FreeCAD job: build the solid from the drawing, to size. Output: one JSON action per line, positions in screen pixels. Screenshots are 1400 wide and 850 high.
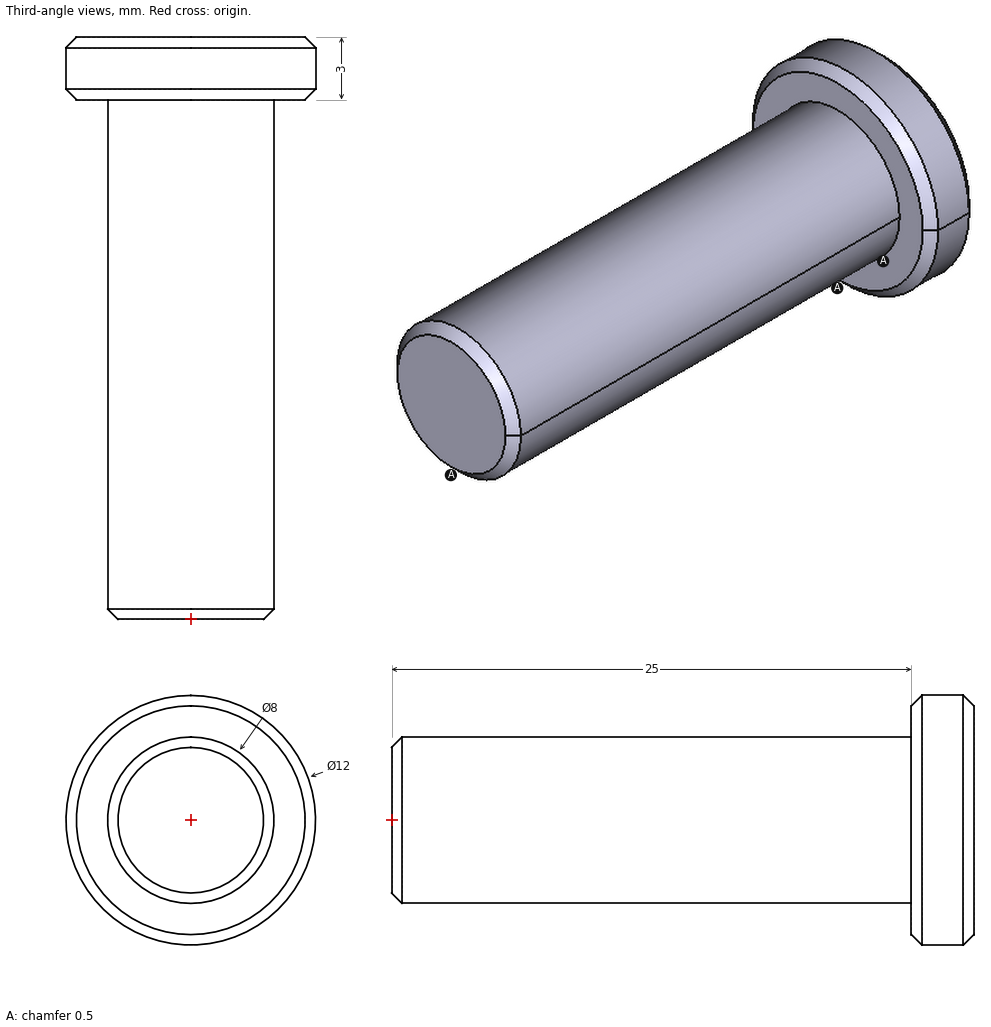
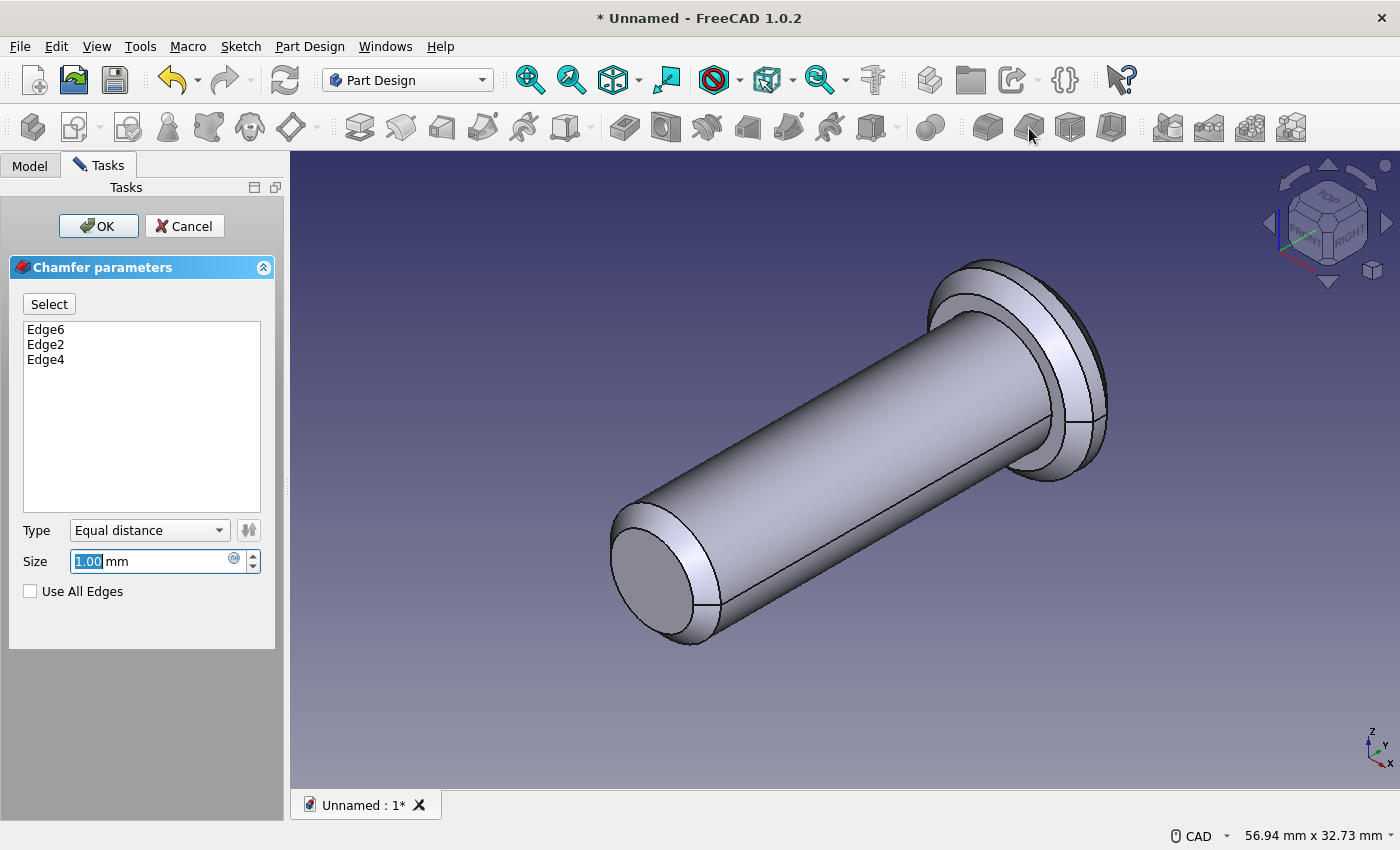
{"action": "type", "text": "0.5"}
{"action": "key", "text": "Tab"}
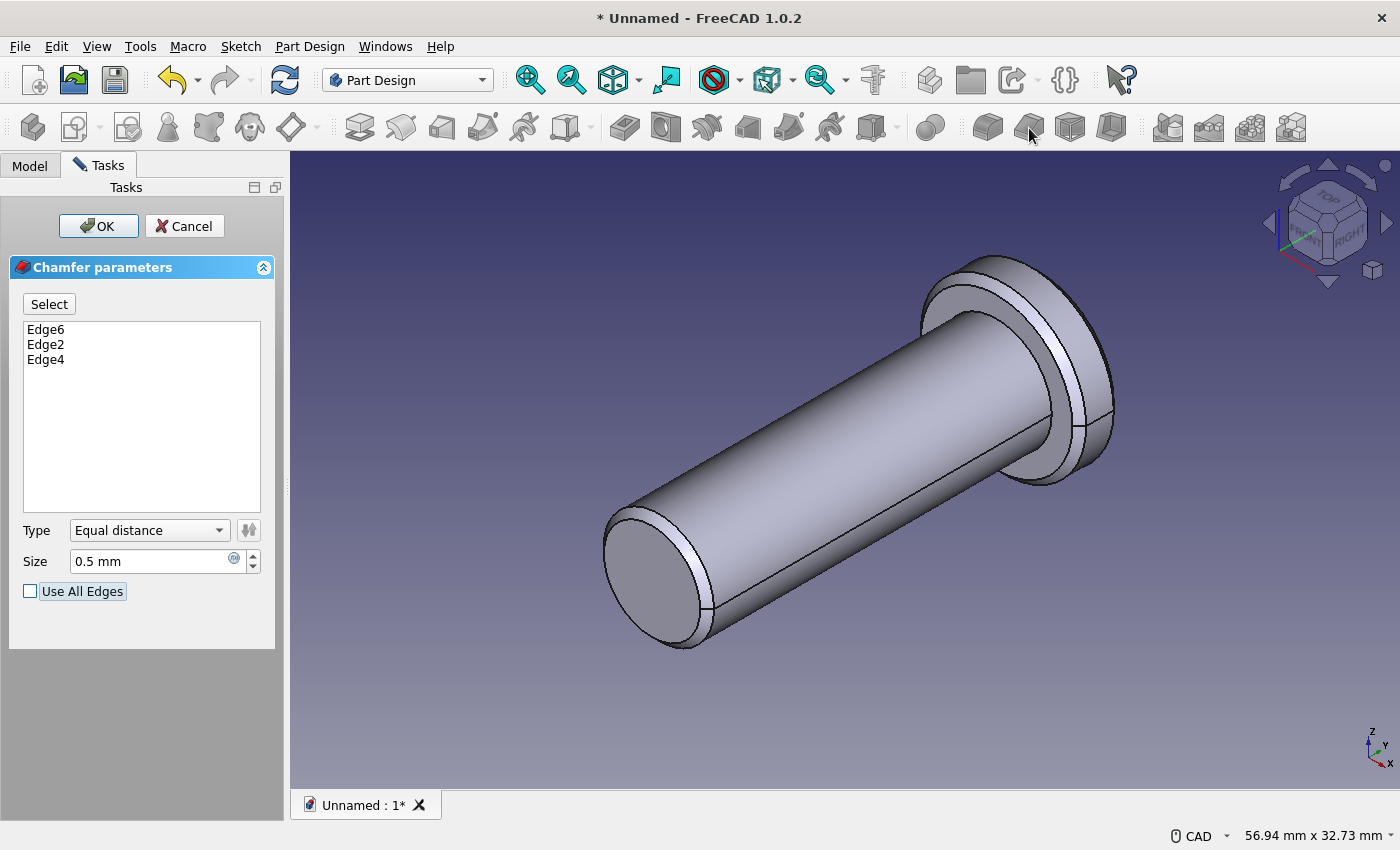
{"action": "left_click", "coordinate": [99, 226]}